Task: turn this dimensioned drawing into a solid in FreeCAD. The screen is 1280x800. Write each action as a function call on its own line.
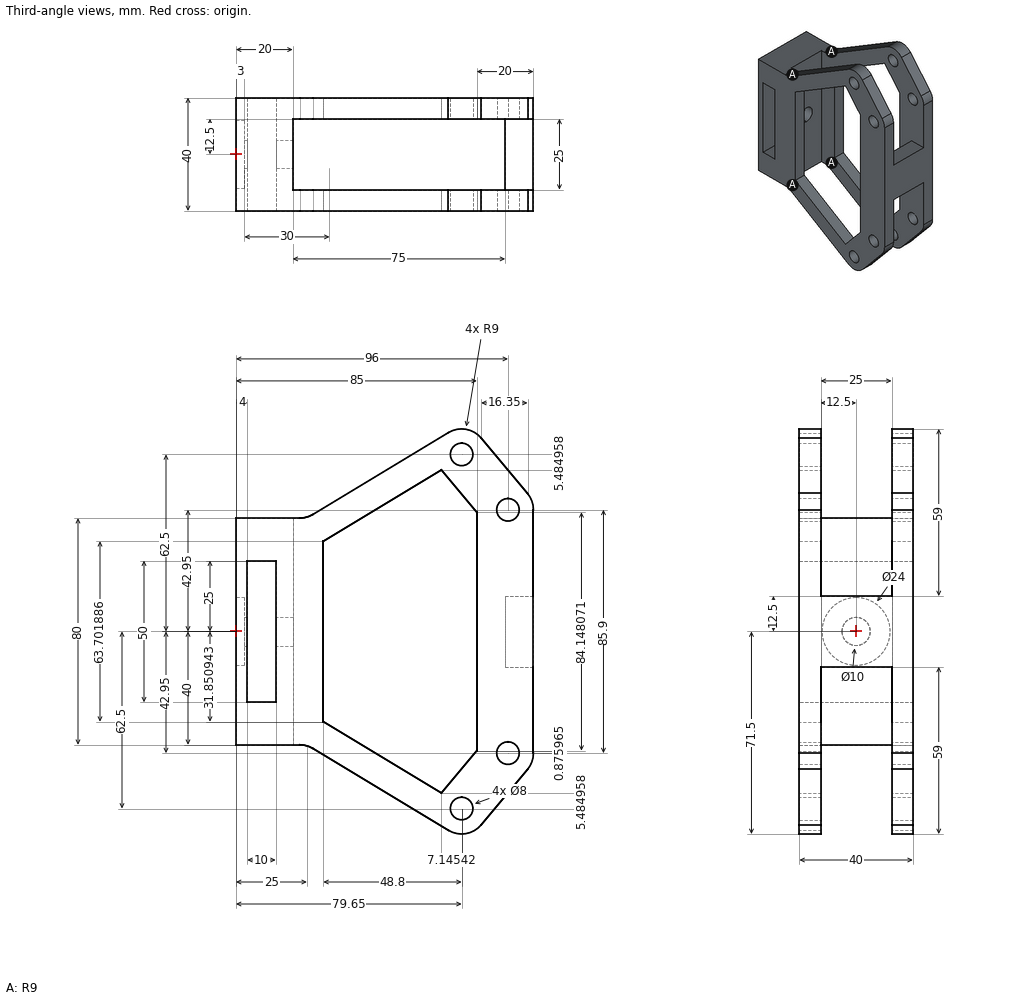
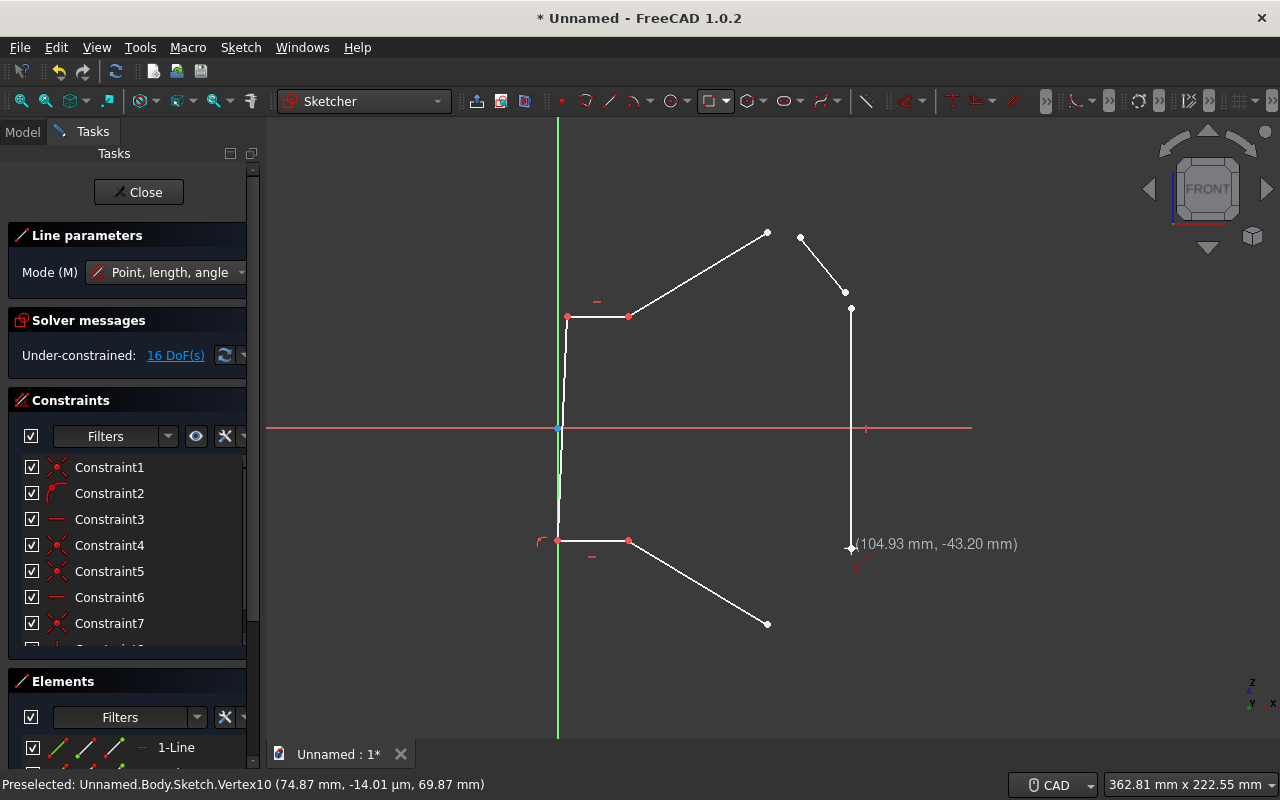
click(845, 564)
click(800, 619)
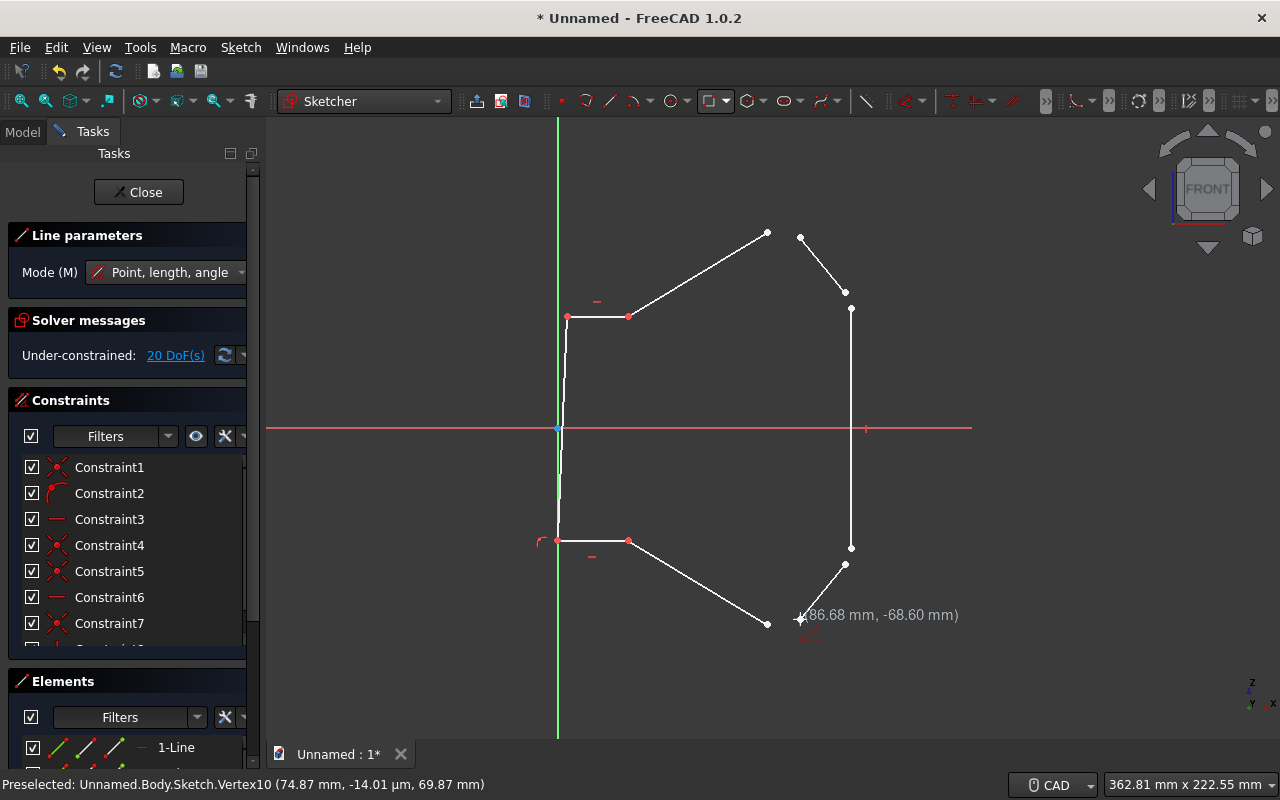
key(g)
key(3)
key(a)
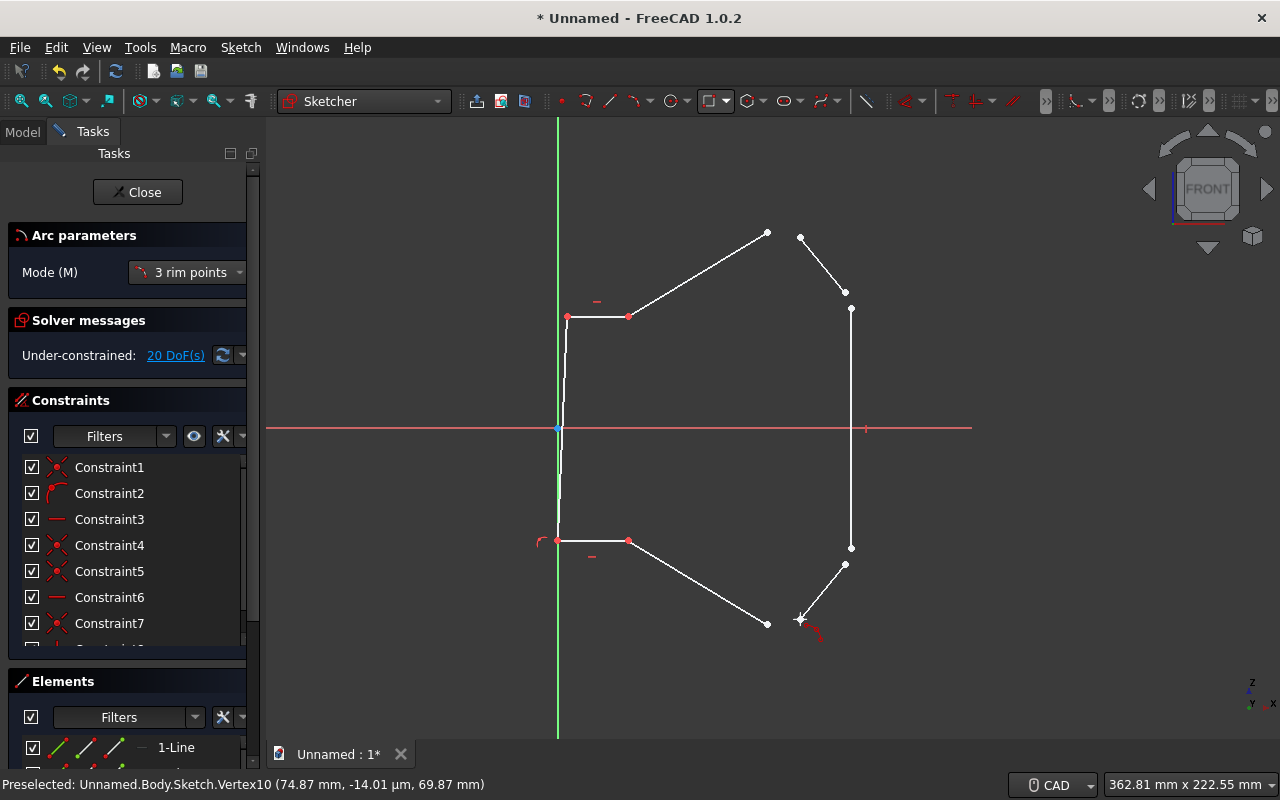
click(767, 233)
click(800, 238)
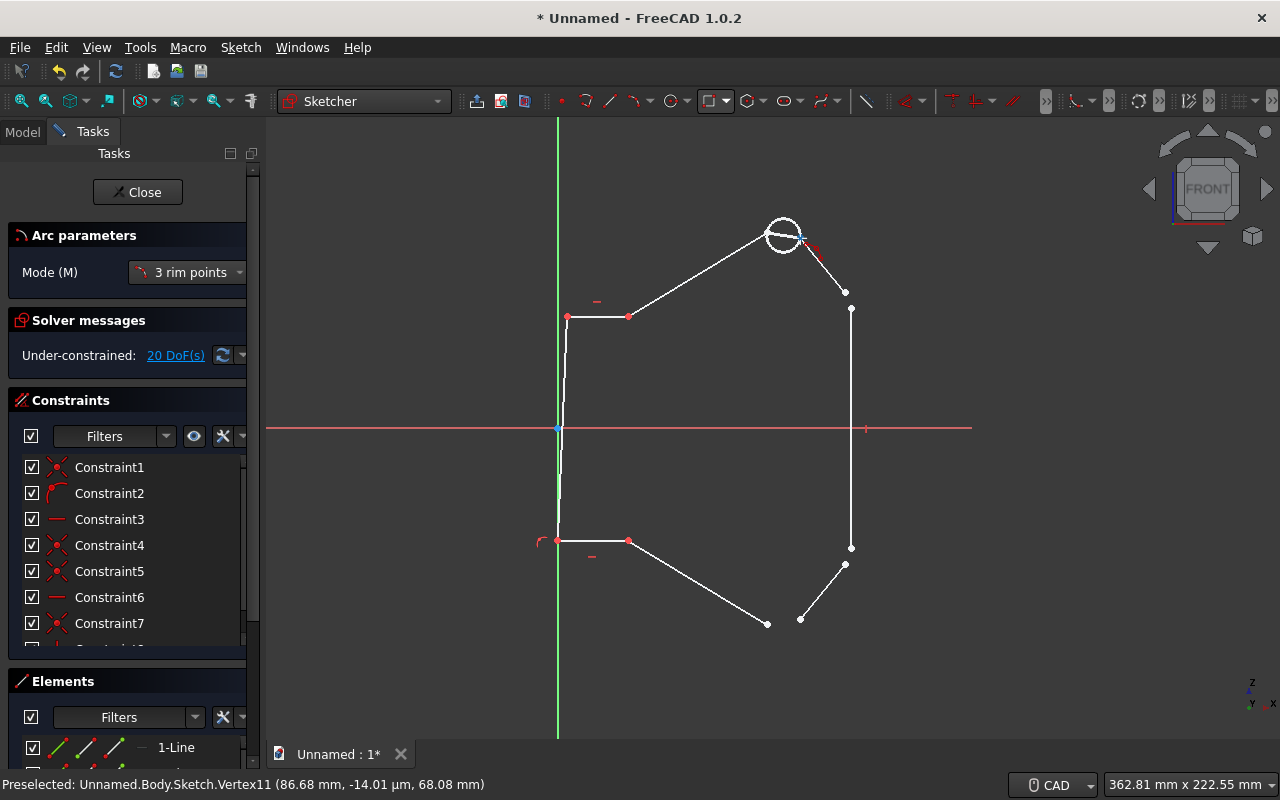
scroll(785, 229, up, 5)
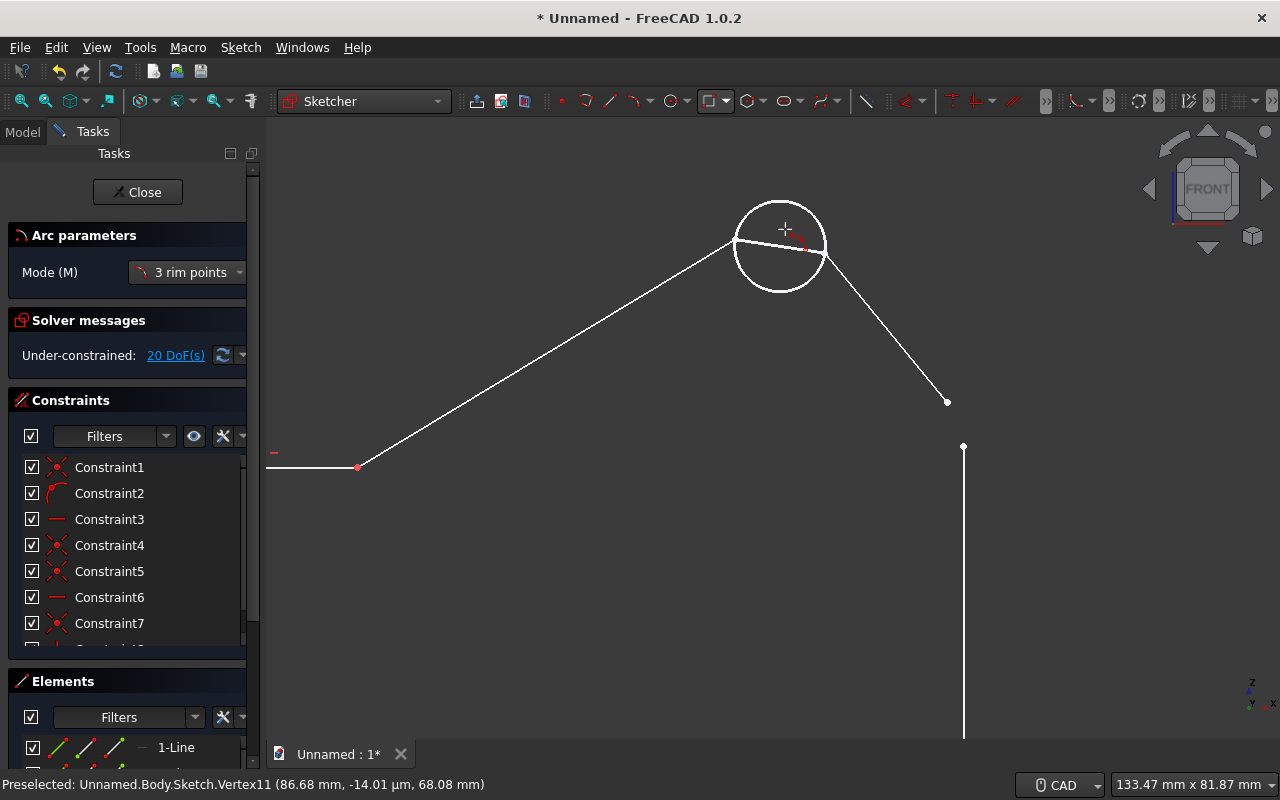
click(783, 228)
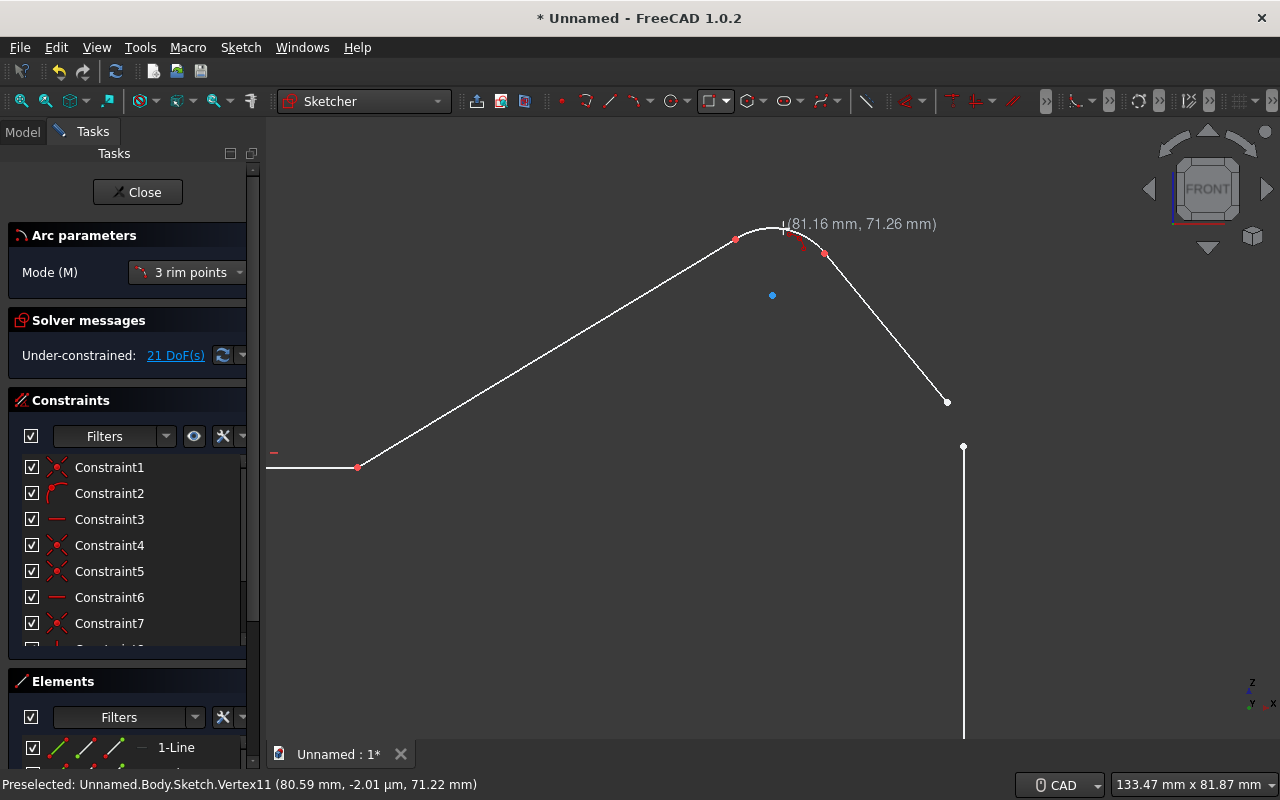
click(947, 403)
click(964, 446)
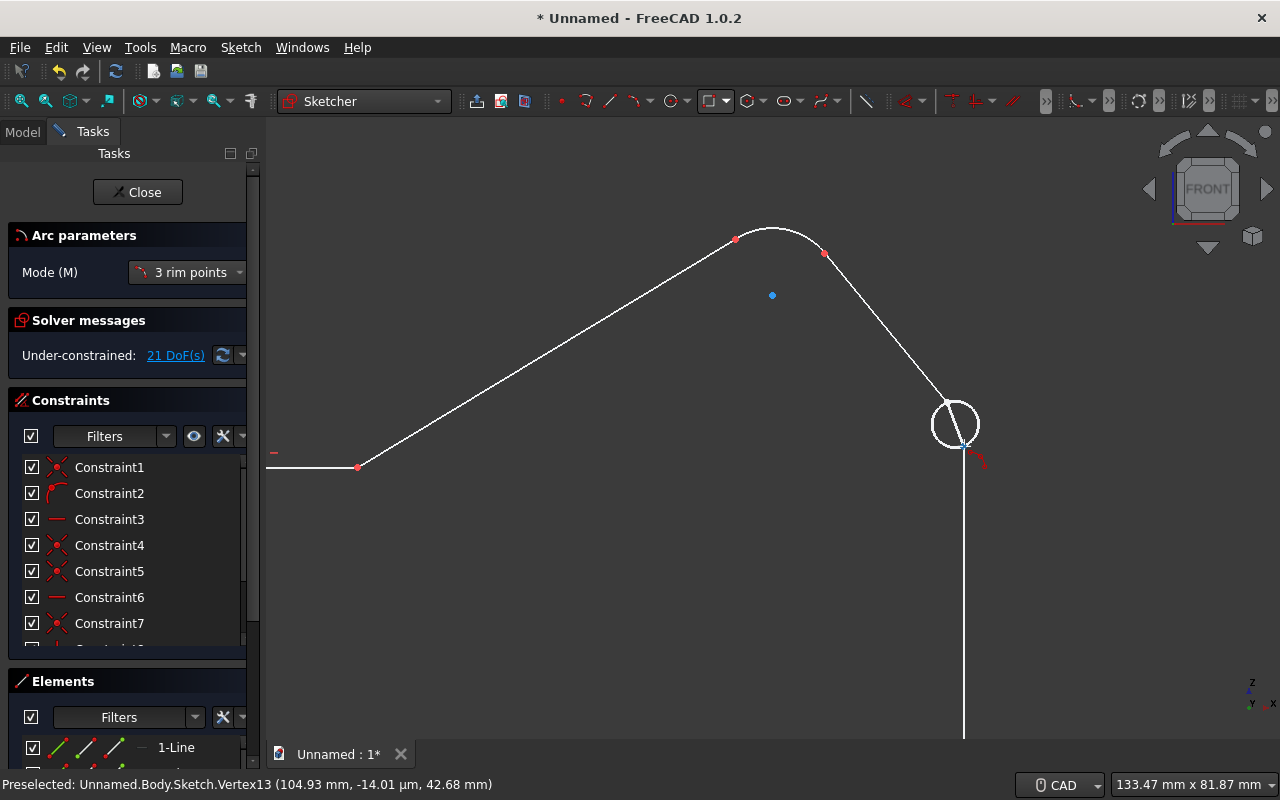
scroll(960, 421, up, 7)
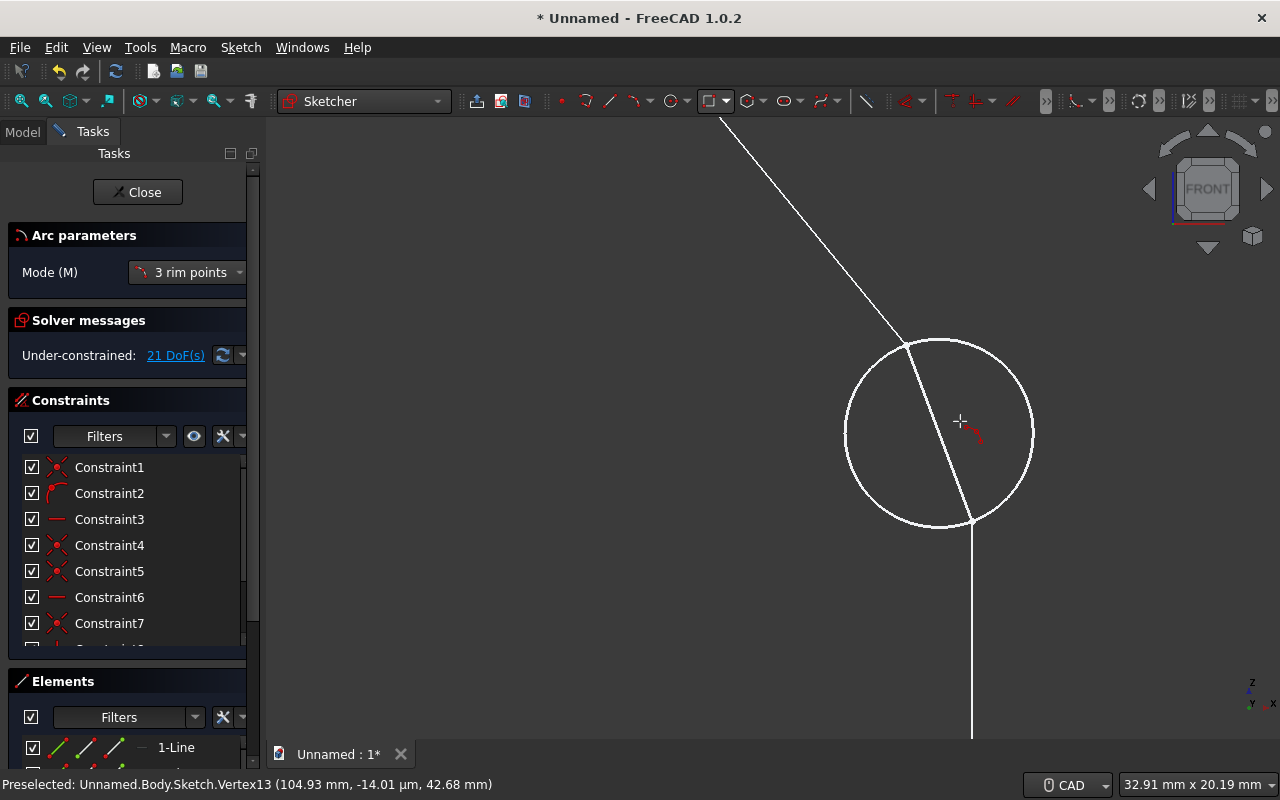
click(958, 418)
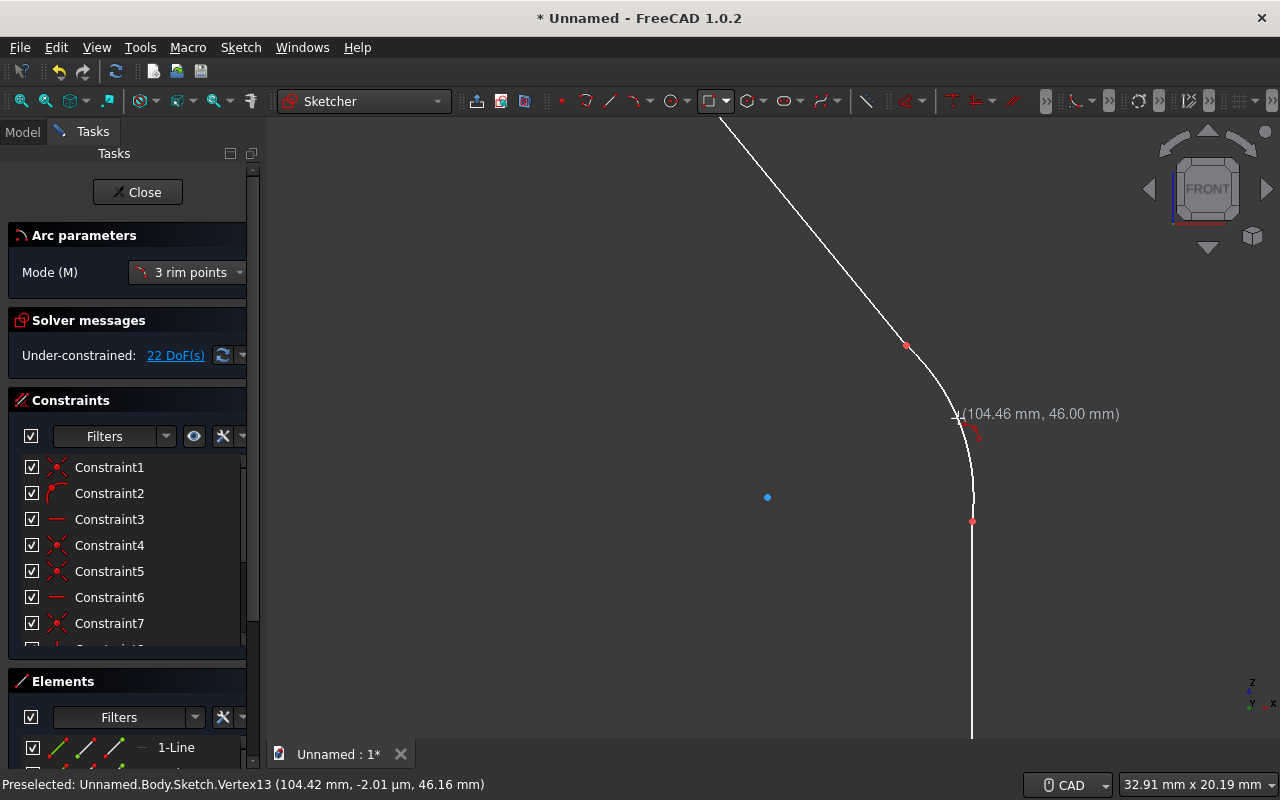
scroll(839, 287, down, 12)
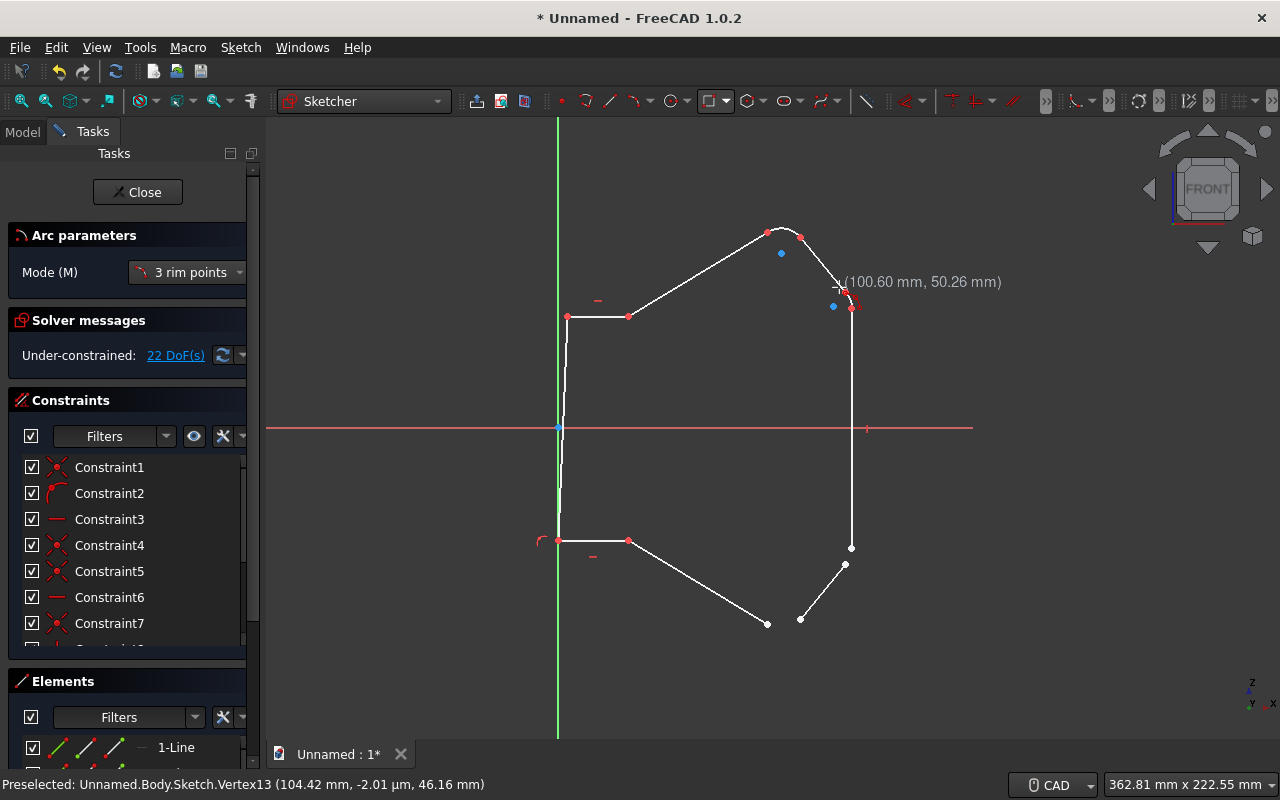
click(852, 549)
click(846, 565)